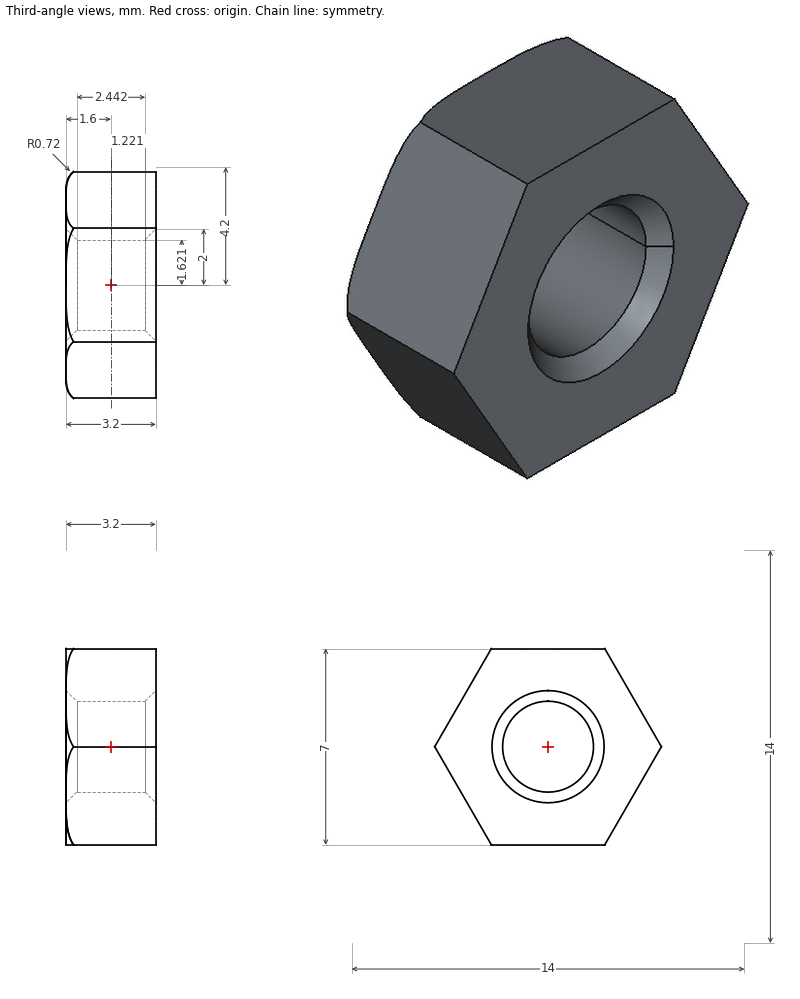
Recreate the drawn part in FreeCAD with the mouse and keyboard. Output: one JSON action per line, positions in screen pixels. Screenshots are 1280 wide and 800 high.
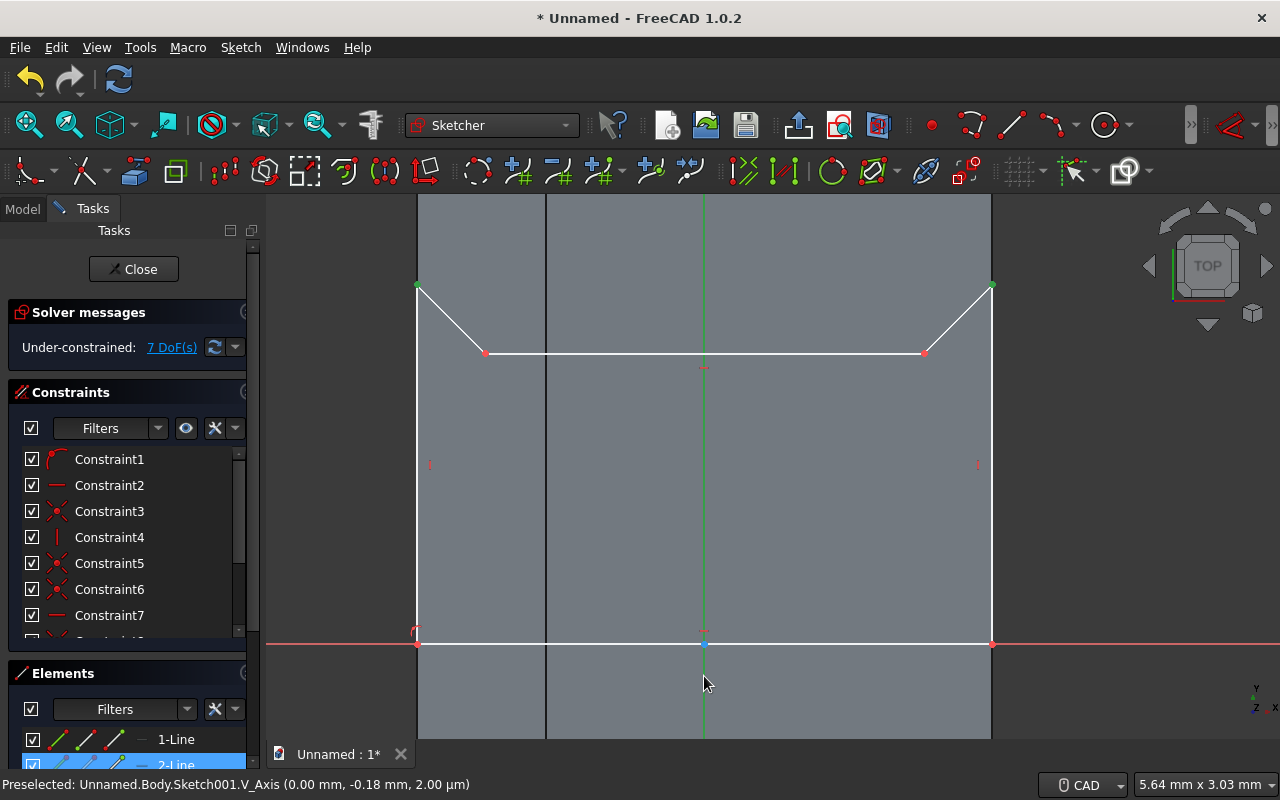
{"action": "key", "text": "s"}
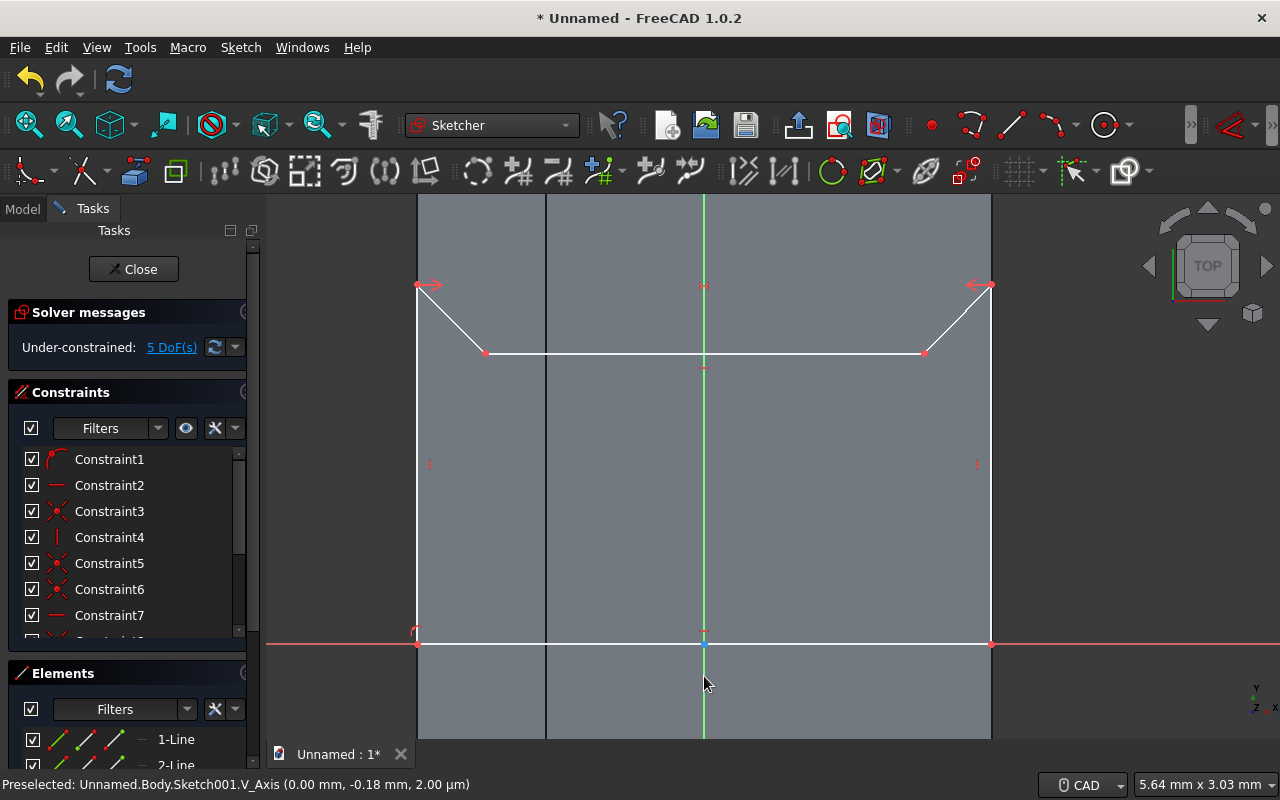
{"action": "key", "text": "d"}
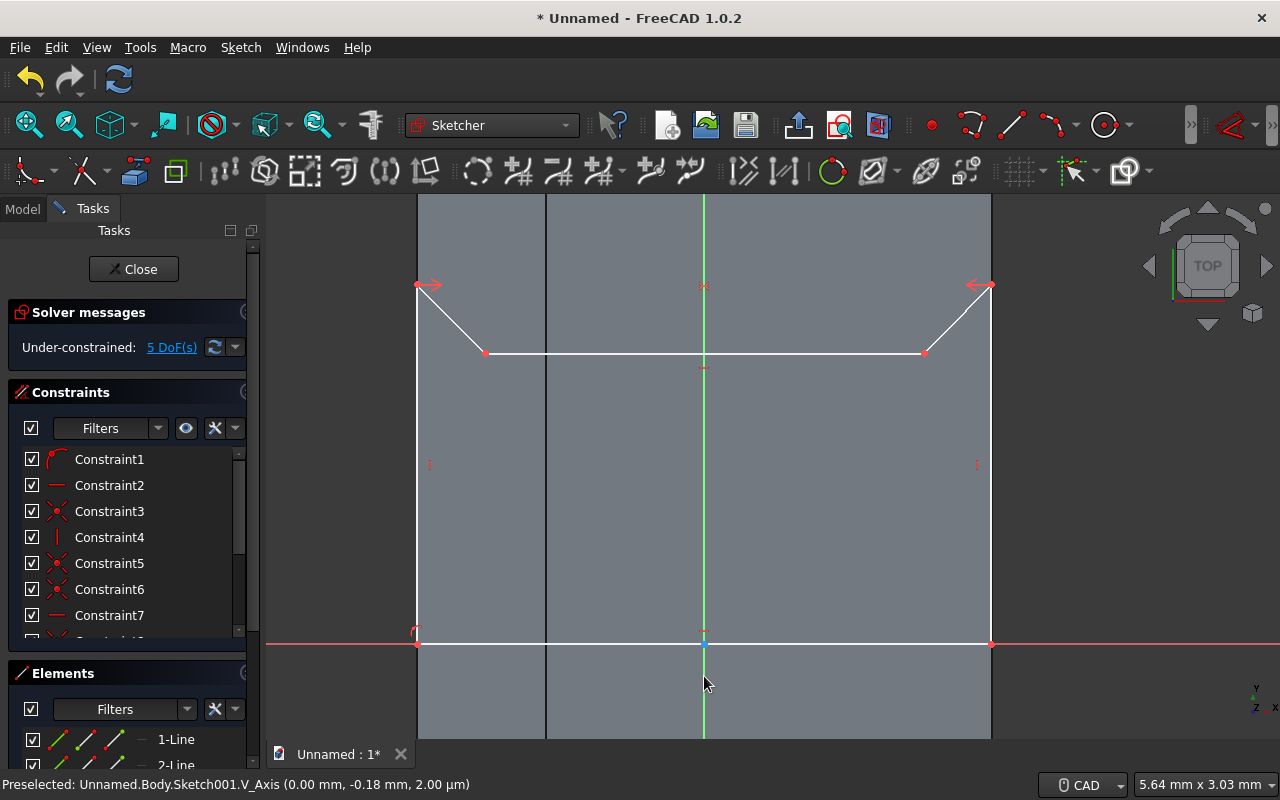
{"action": "left_click", "coordinate": [991, 536]}
{"action": "left_click", "coordinate": [1025, 465]}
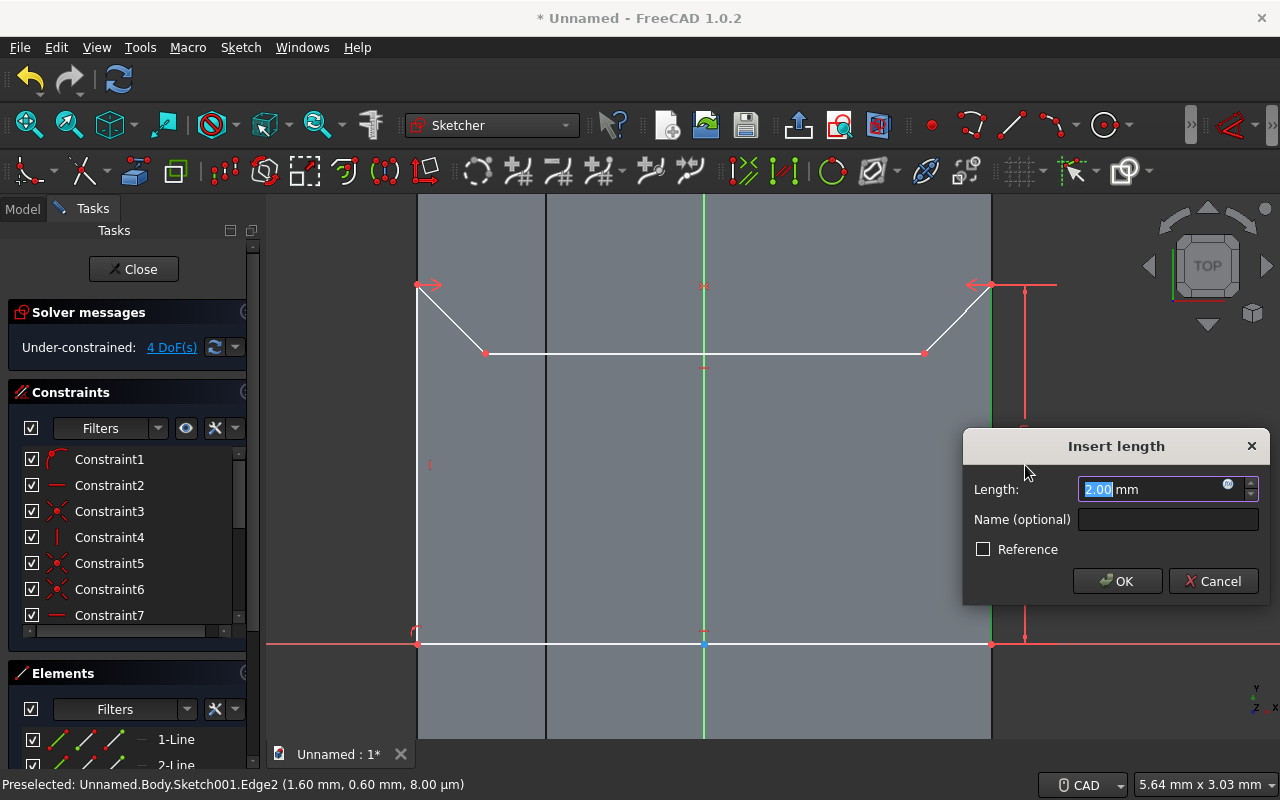
{"action": "type", "text": "2"}
{"action": "key", "text": "Return"}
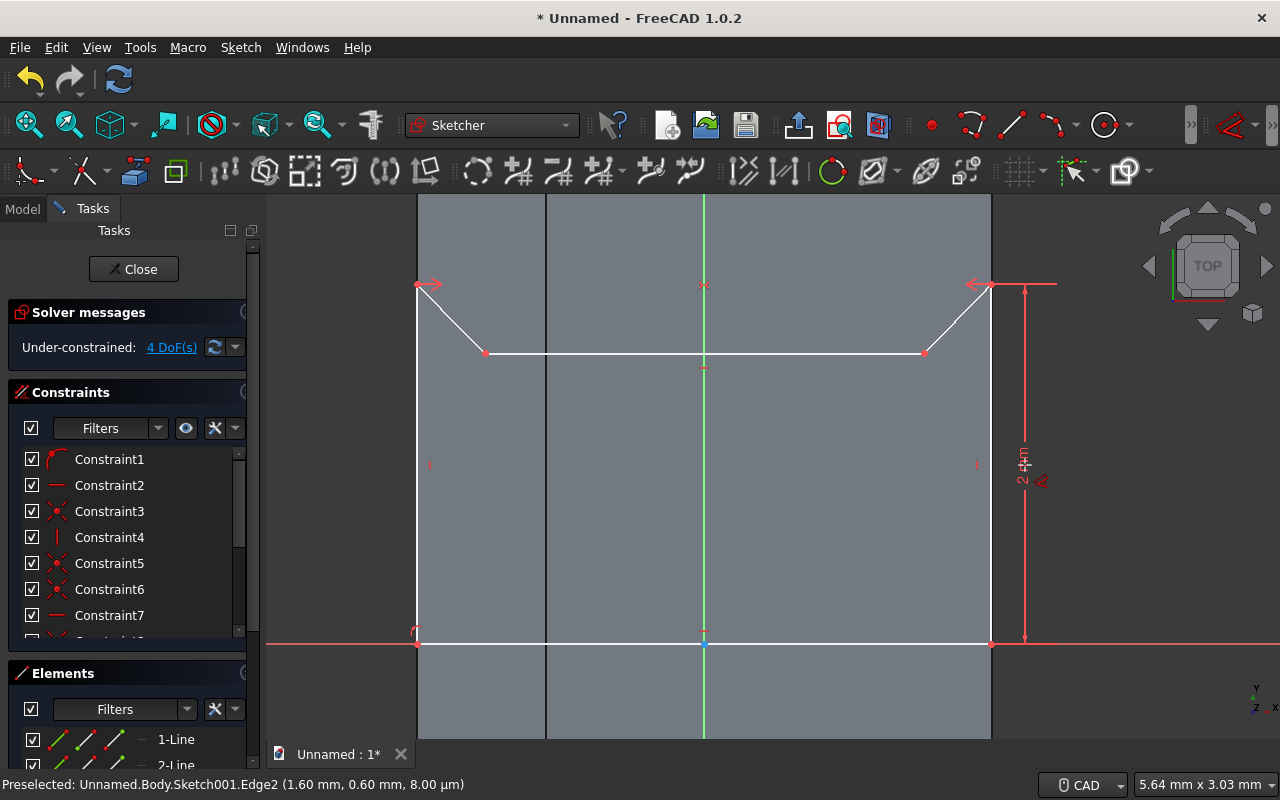
{"action": "left_click", "coordinate": [589, 644]}
{"action": "left_click", "coordinate": [572, 678]}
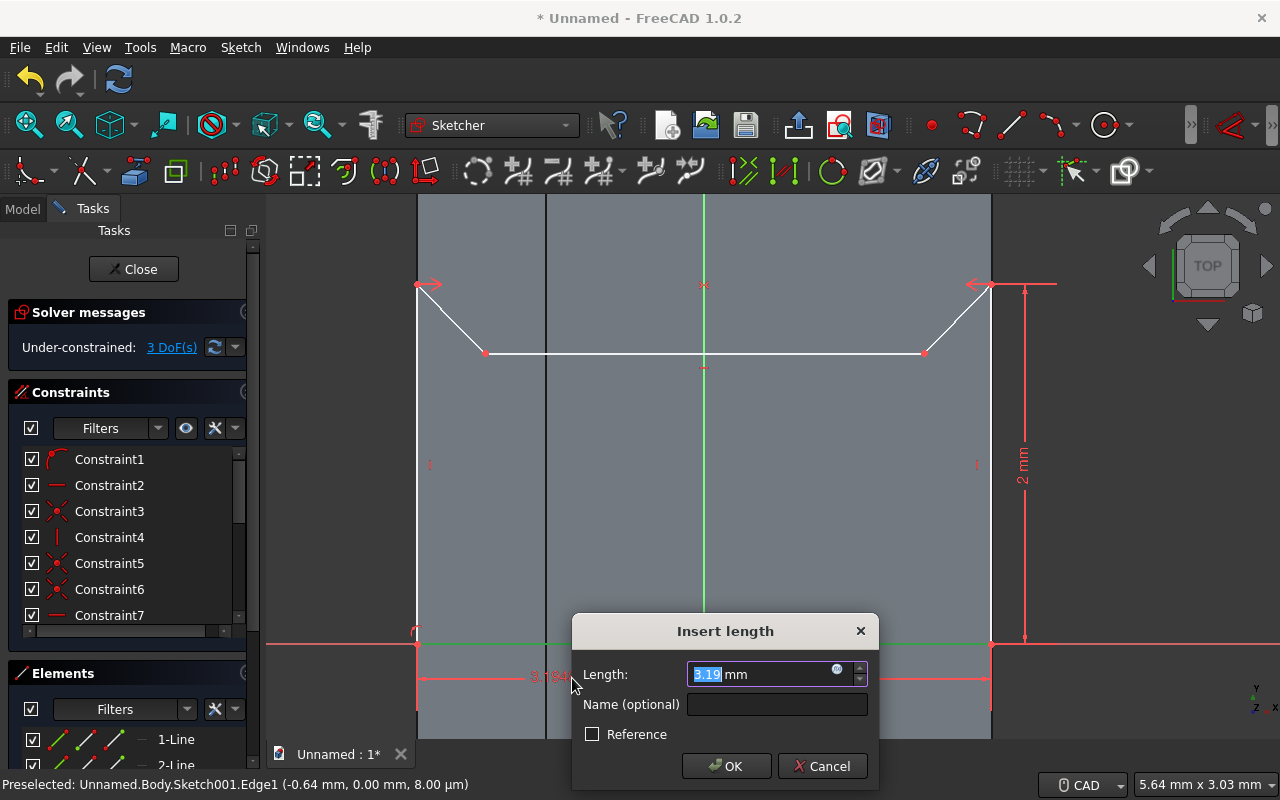
{"action": "type", "text": "3.2"}
{"action": "key", "text": "Return"}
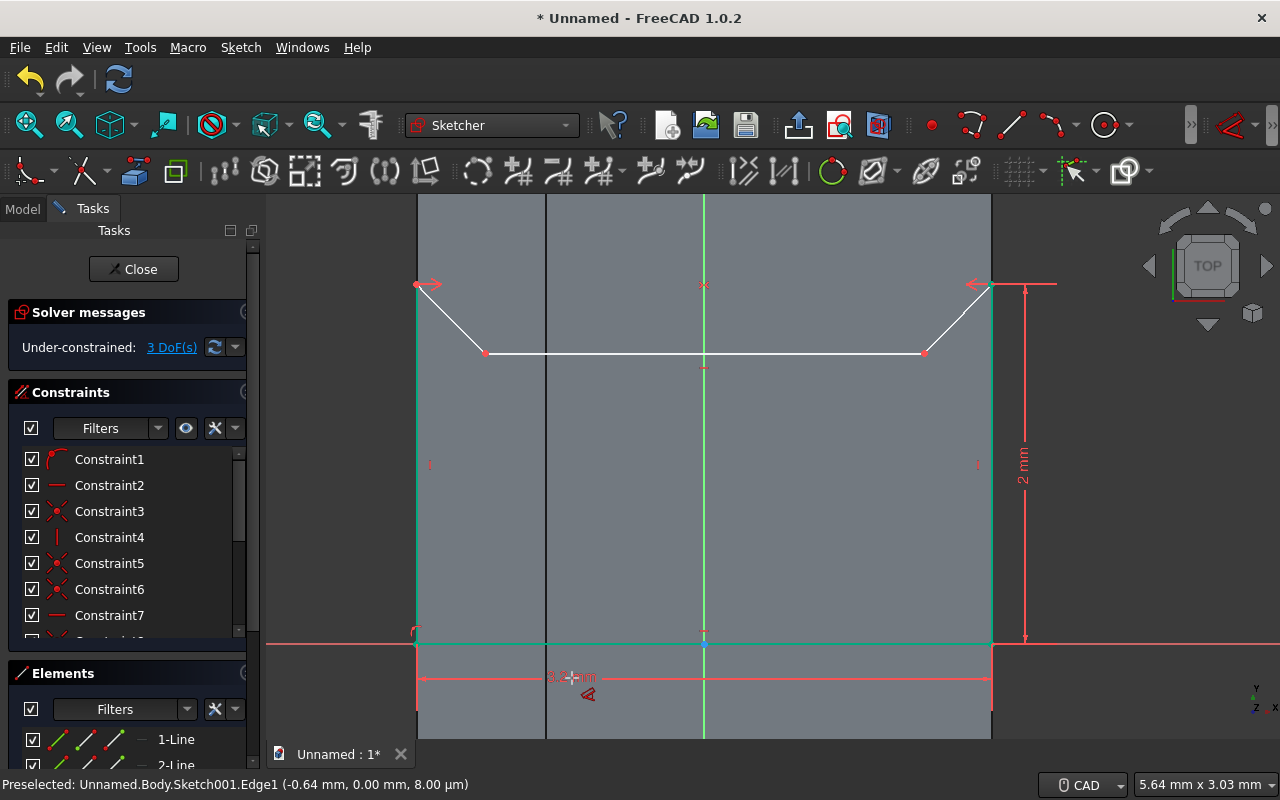
{"action": "left_click", "coordinate": [792, 354]}
{"action": "left_click", "coordinate": [604, 320]}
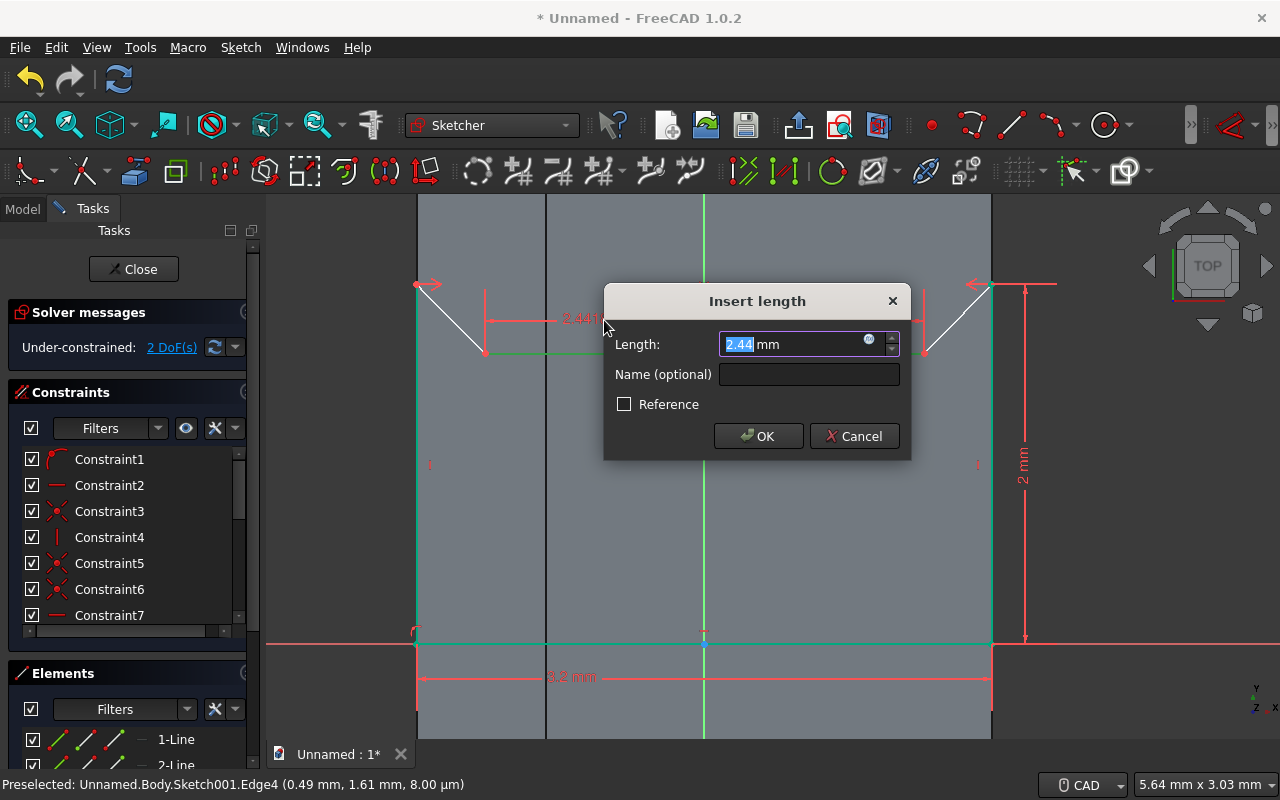
{"action": "type", "text": "2.442"}
{"action": "key", "text": "Return"}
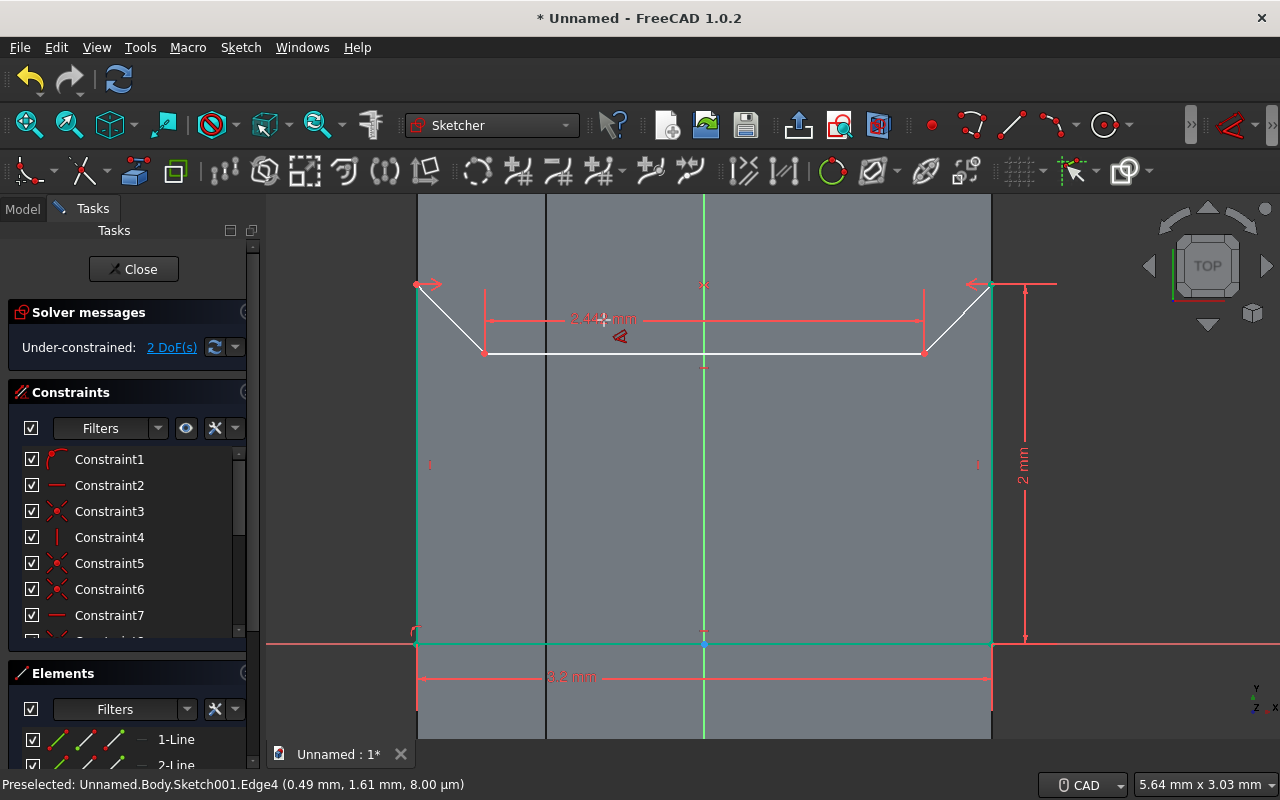
{"action": "left_click", "coordinate": [924, 354]}
{"action": "left_click", "coordinate": [814, 678]}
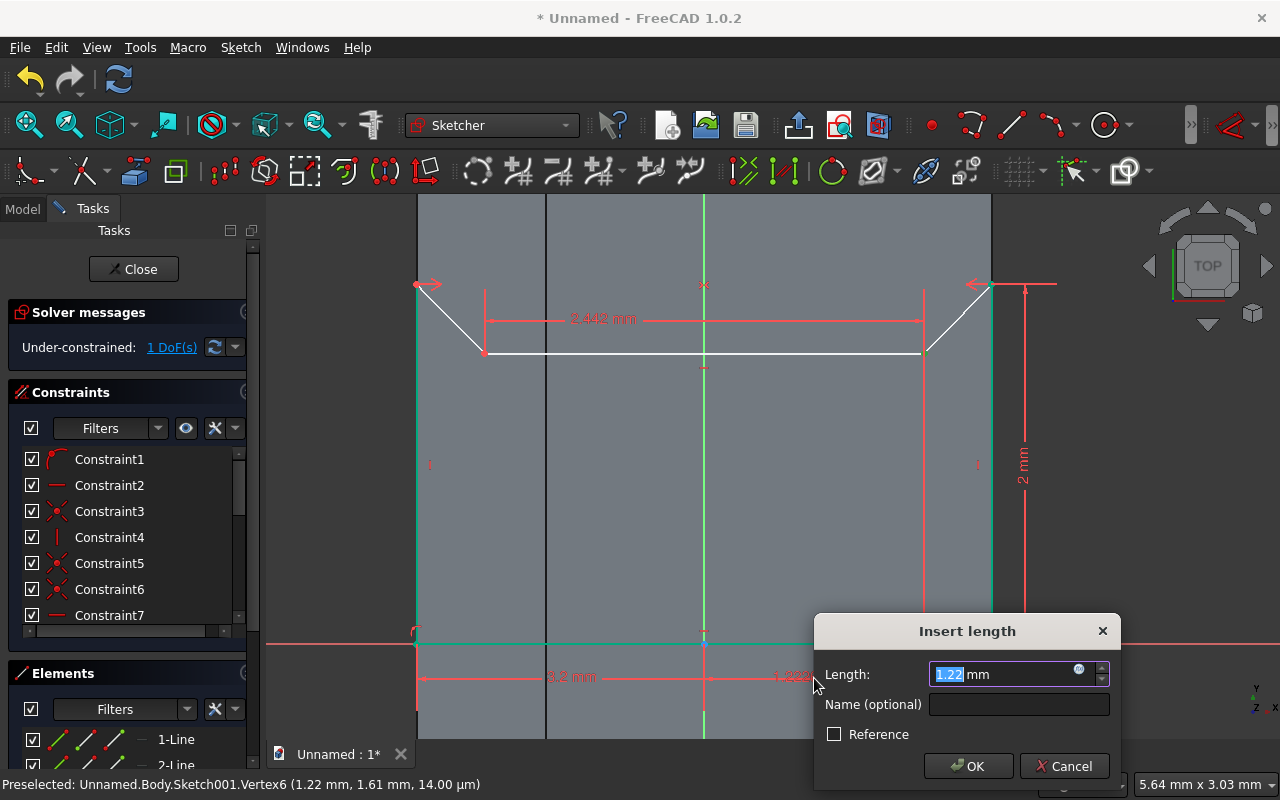
{"action": "type", "text": "1.221"}
{"action": "key", "text": "Return"}